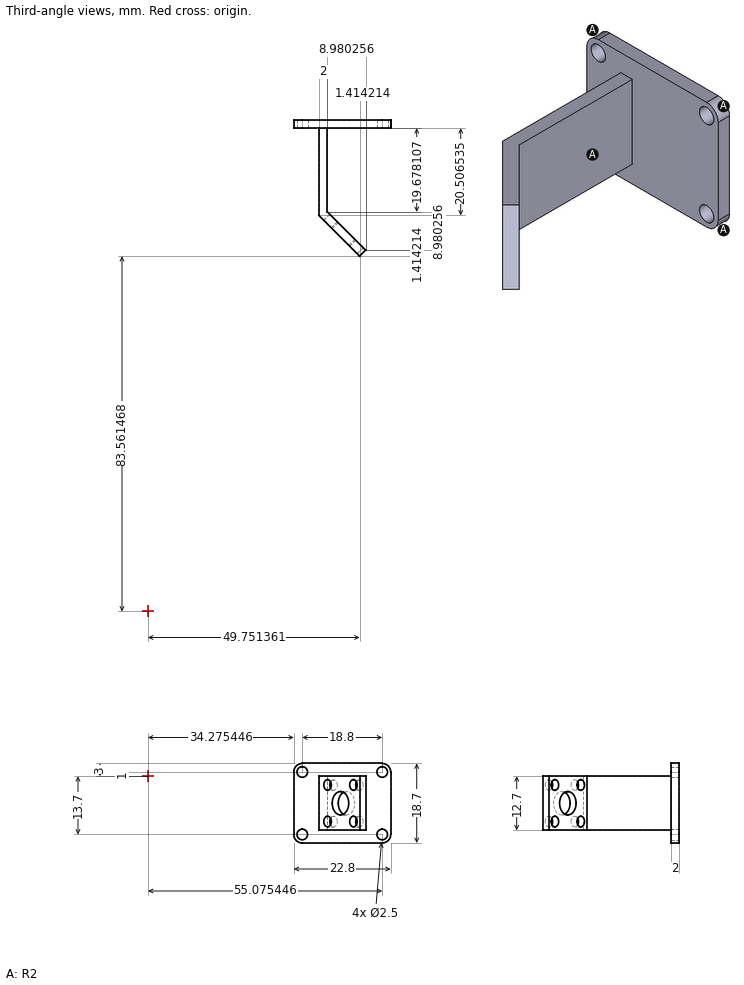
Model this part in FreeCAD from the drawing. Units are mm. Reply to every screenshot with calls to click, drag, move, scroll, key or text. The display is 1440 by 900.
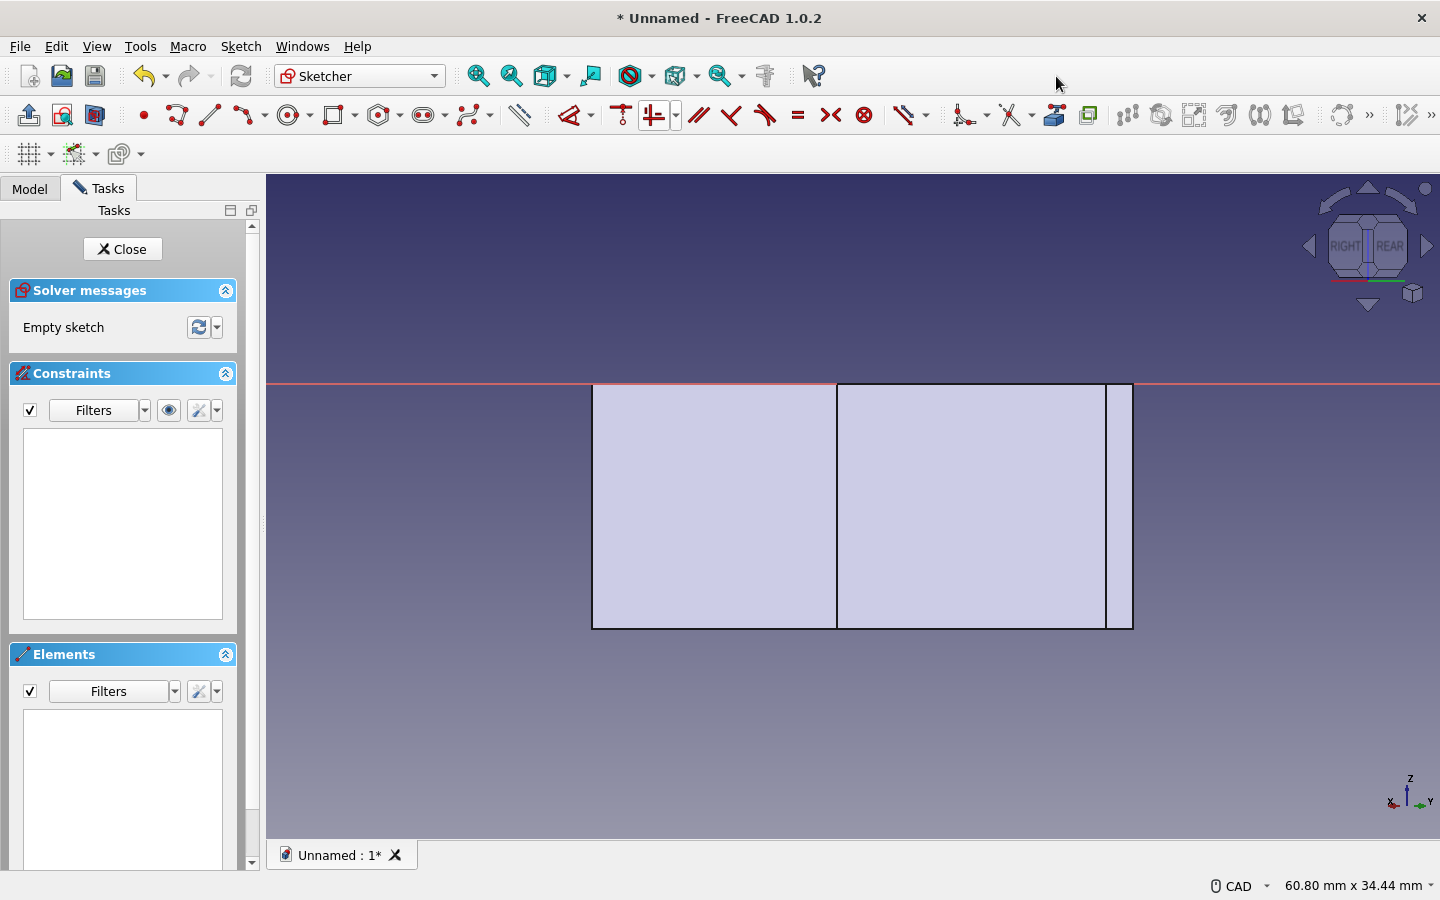
scroll(692, 506, up, 7)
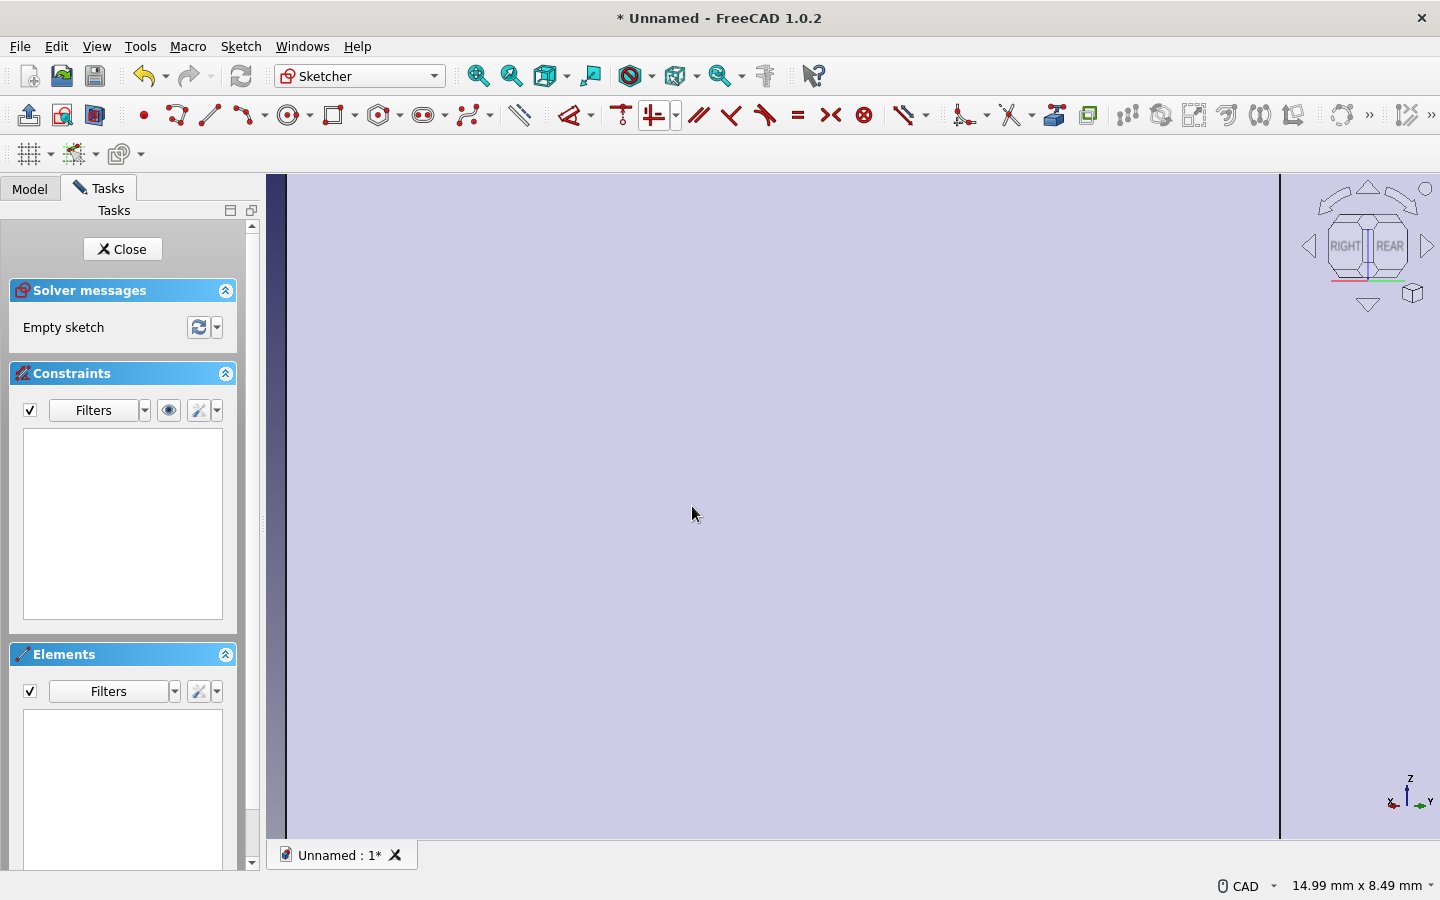
click(288, 116)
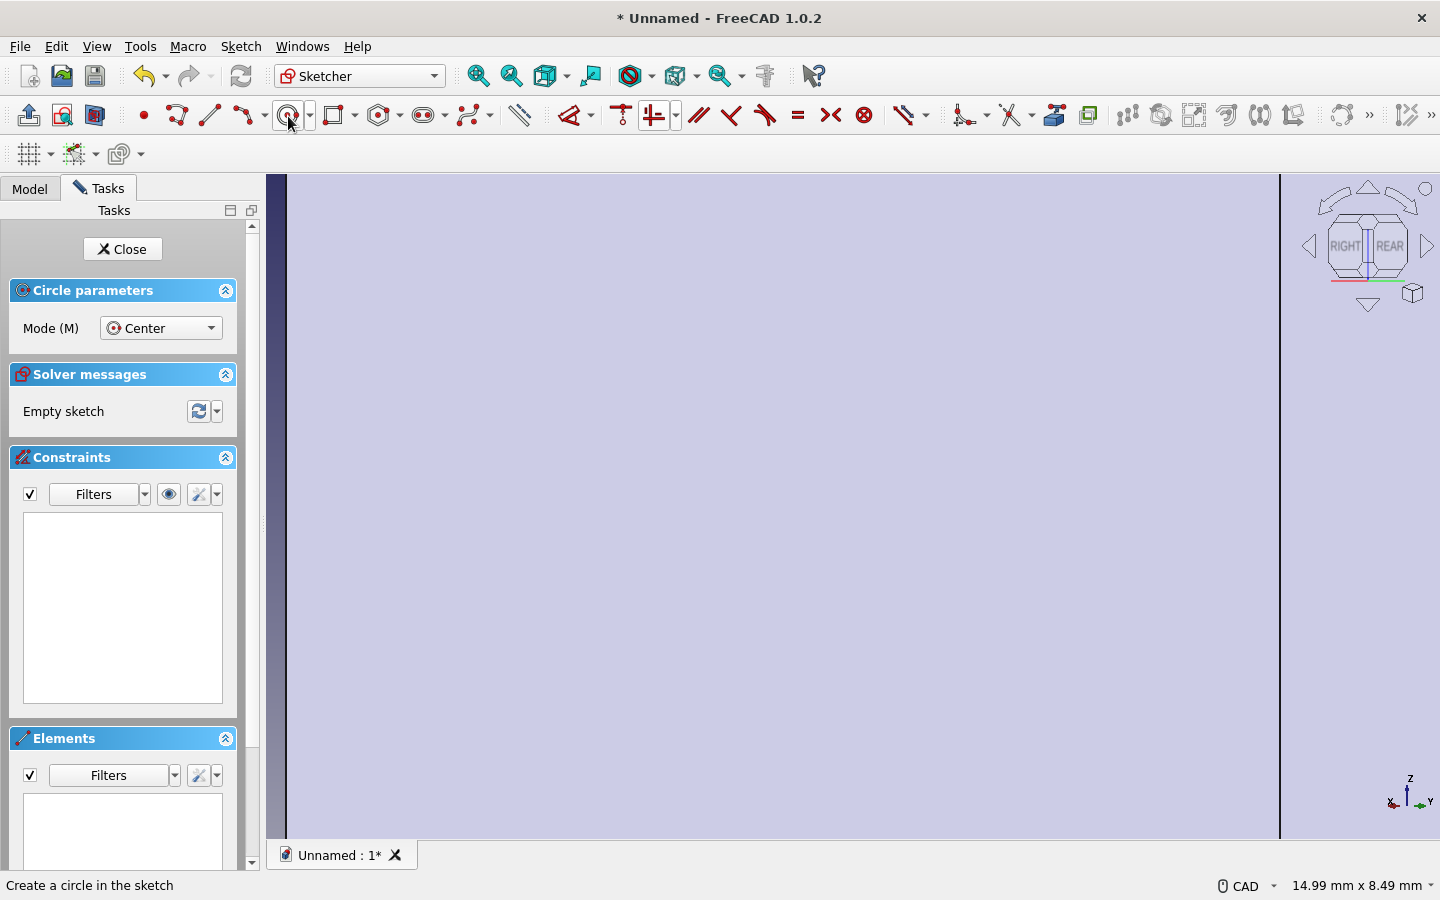
click(783, 506)
move(935, 354)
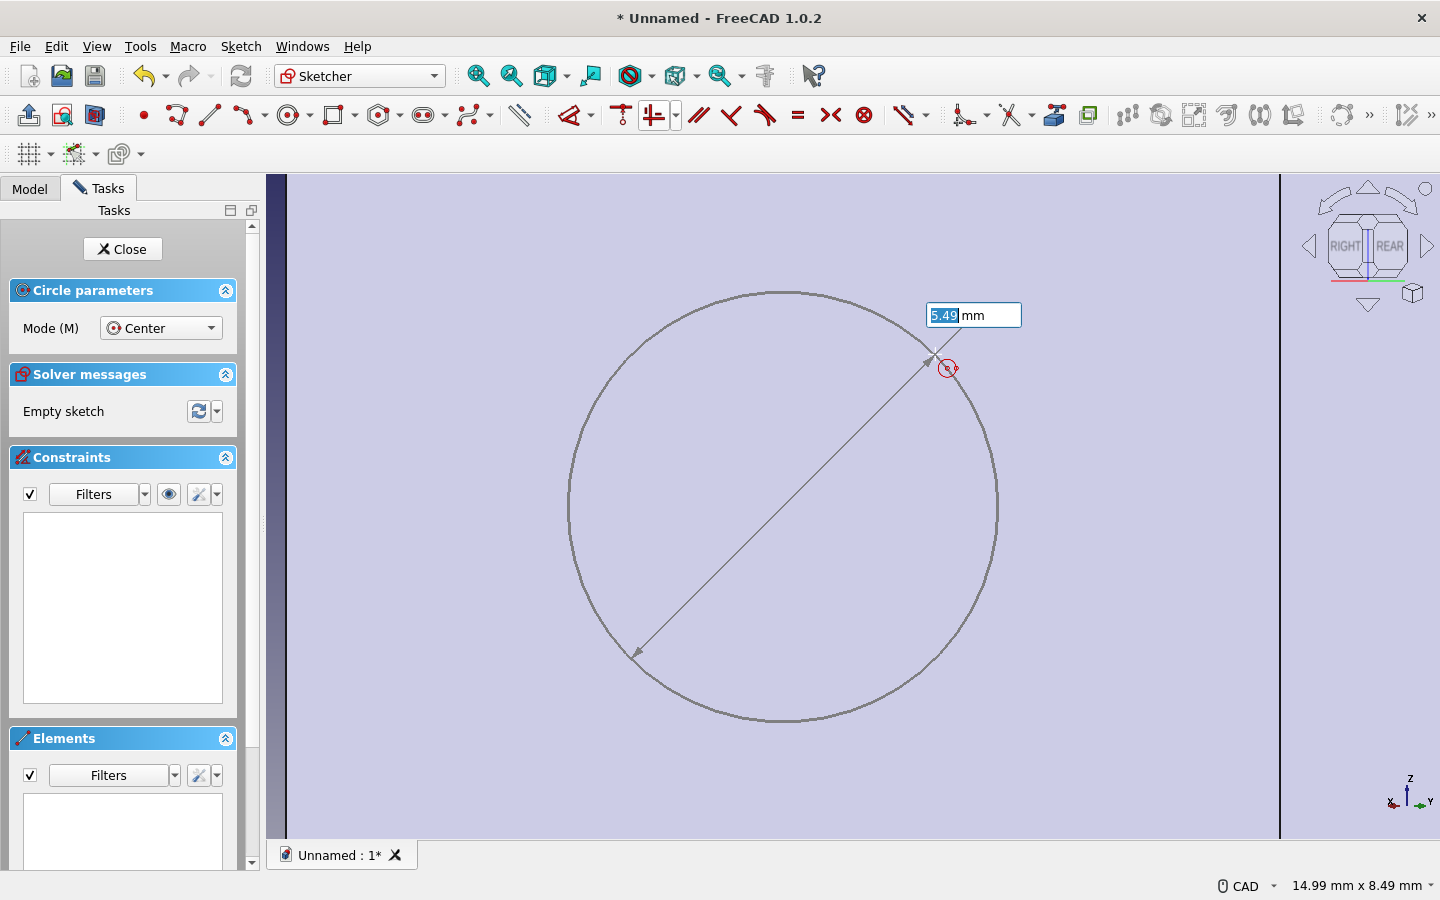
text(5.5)
key(Return)
key(Escape)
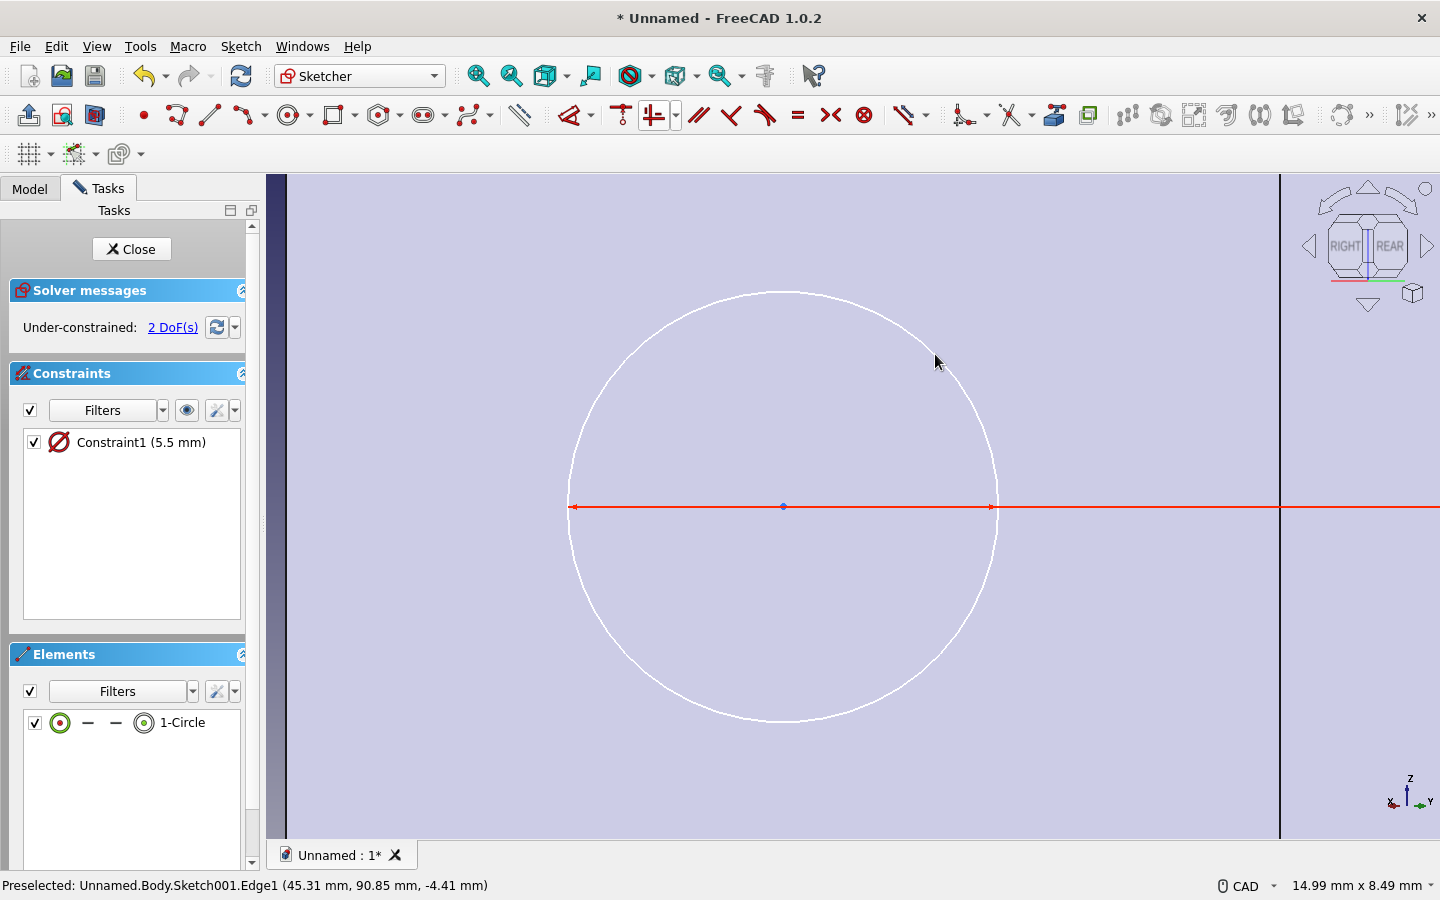
key(d)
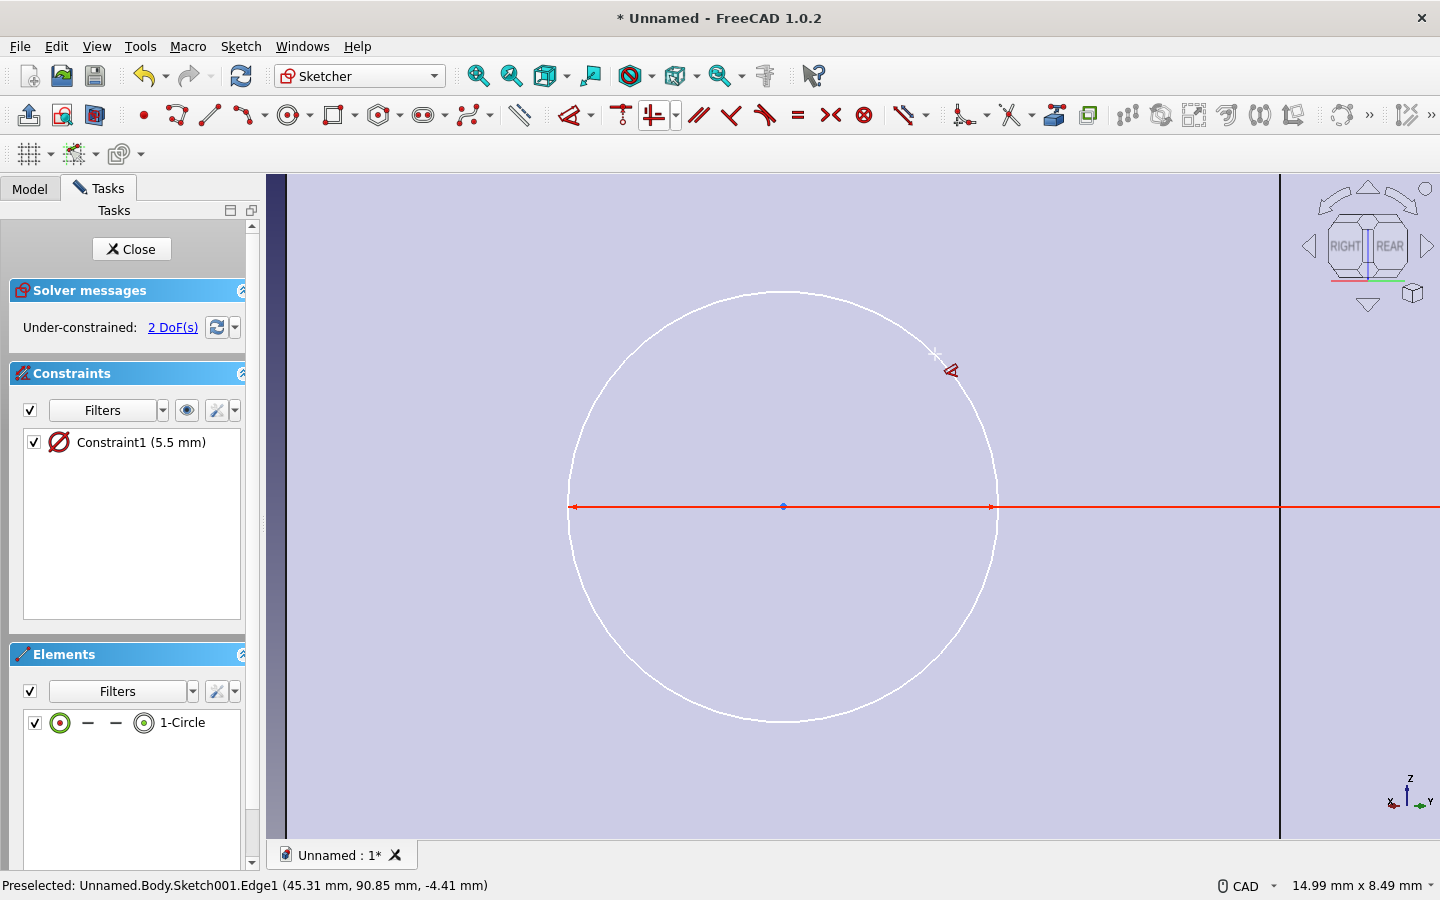
click(783, 507)
click(817, 355)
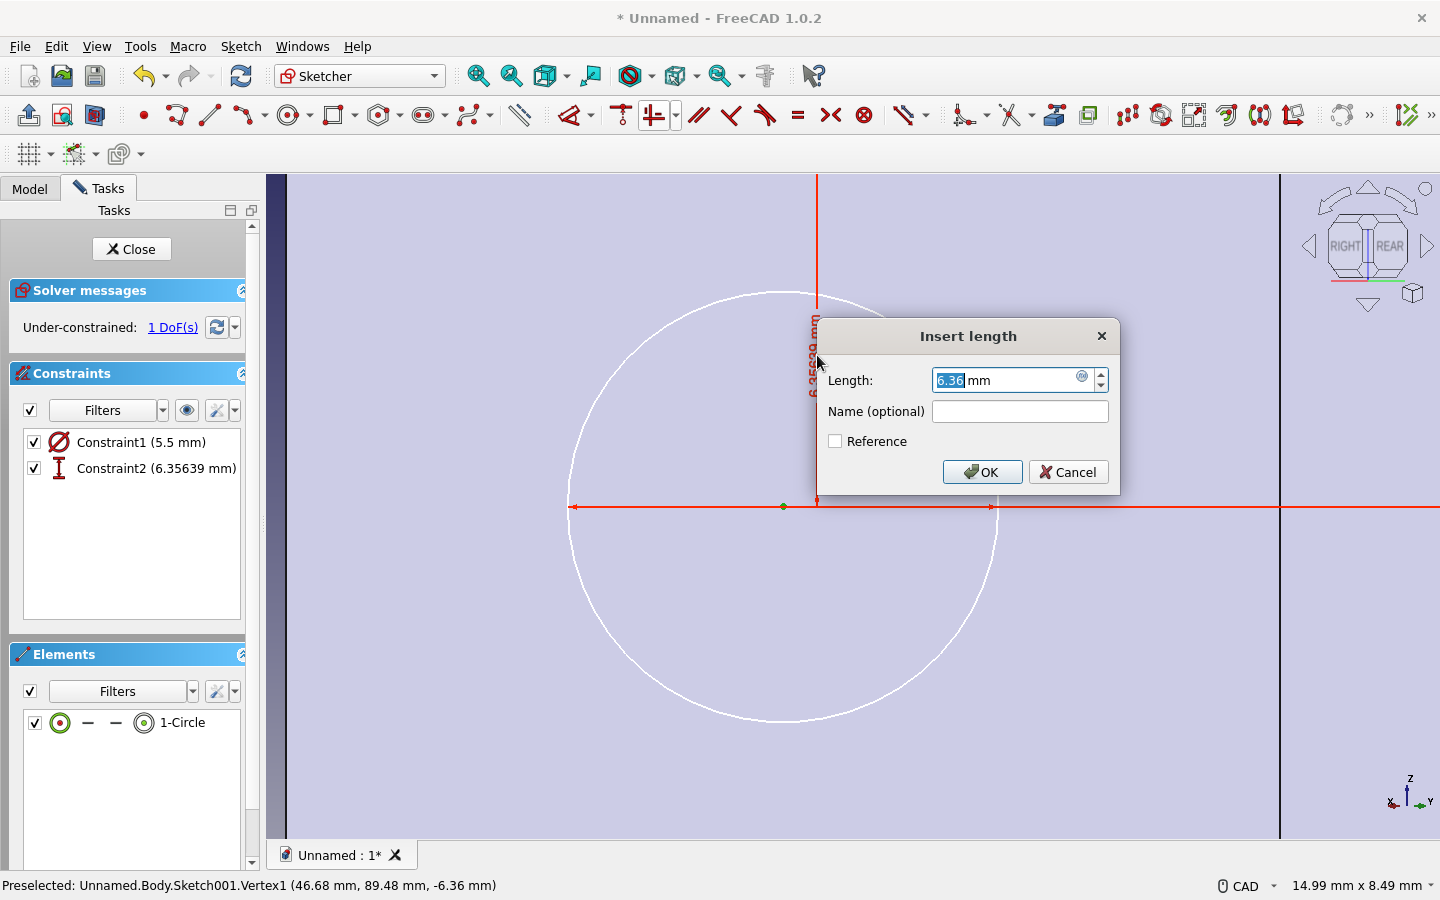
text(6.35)
key(Return)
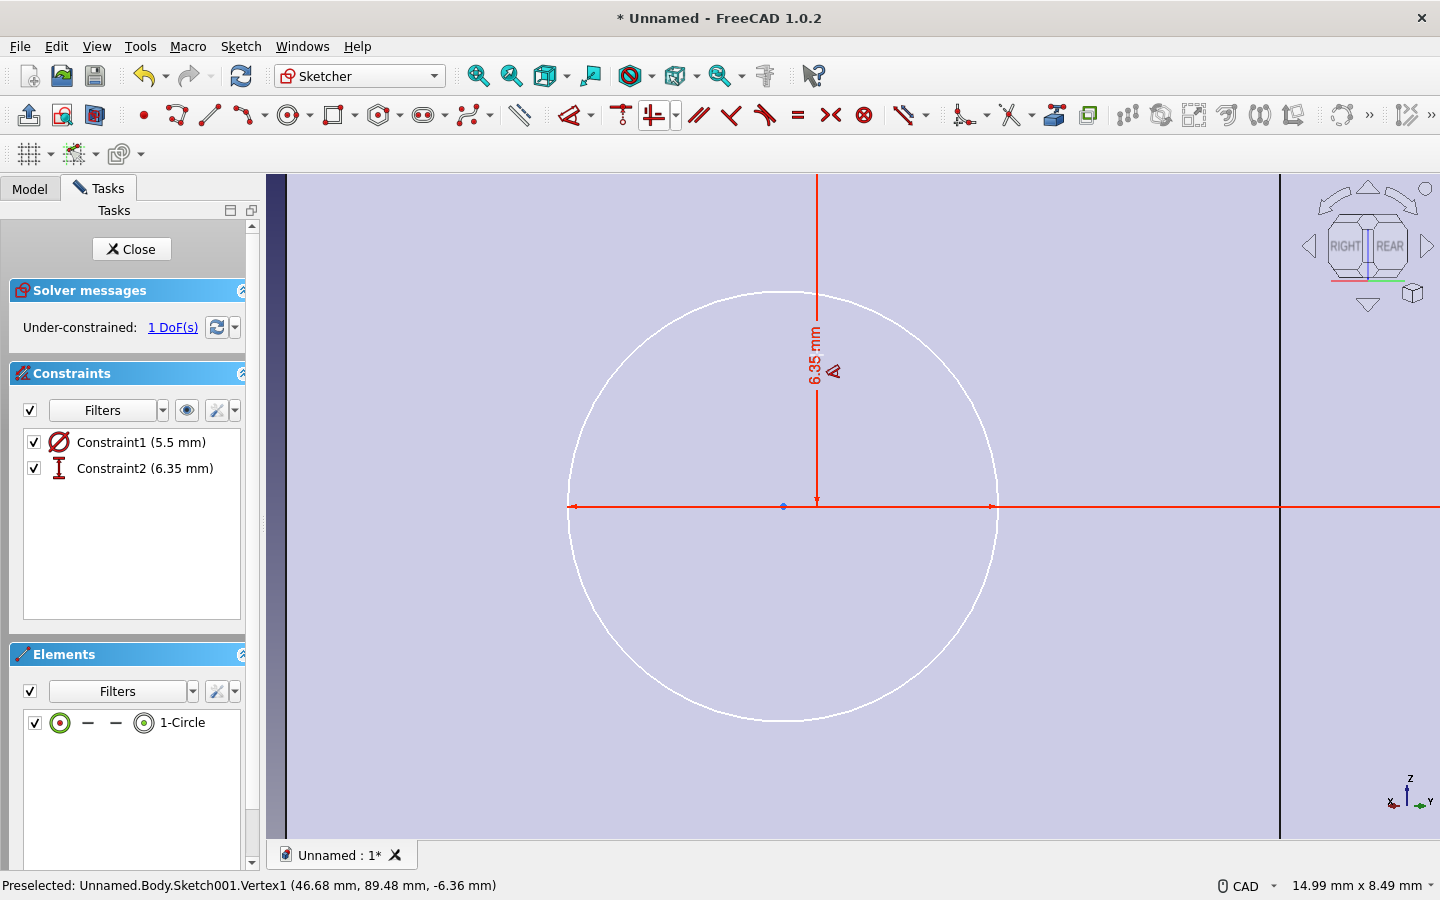
click(783, 506)
click(538, 540)